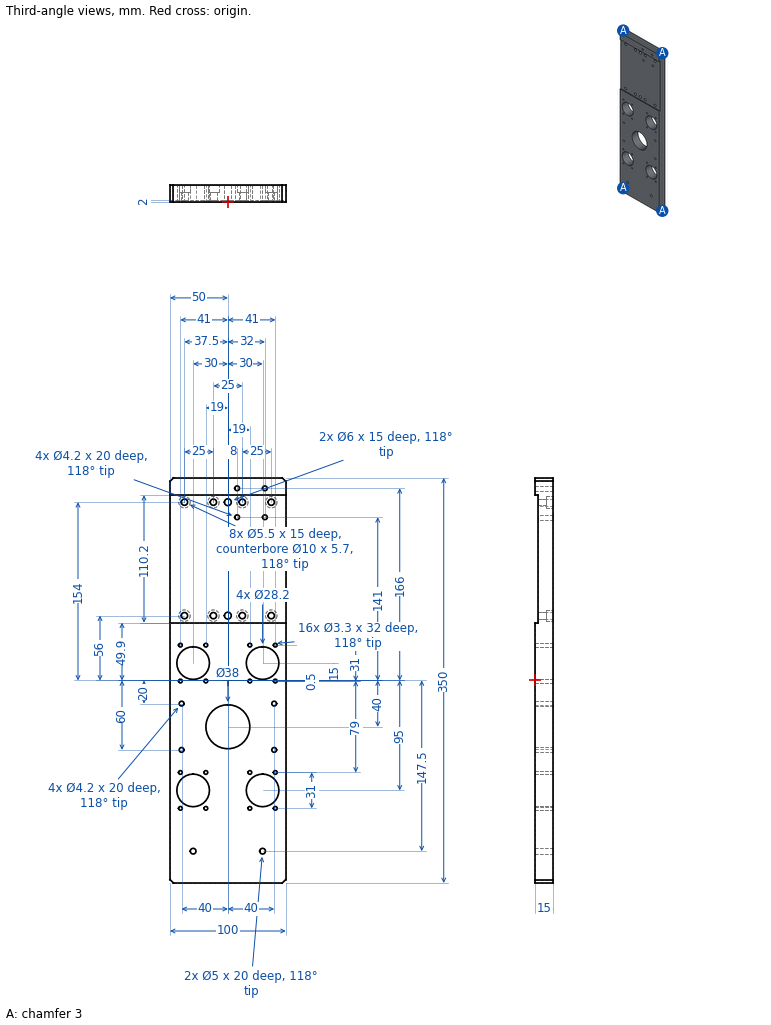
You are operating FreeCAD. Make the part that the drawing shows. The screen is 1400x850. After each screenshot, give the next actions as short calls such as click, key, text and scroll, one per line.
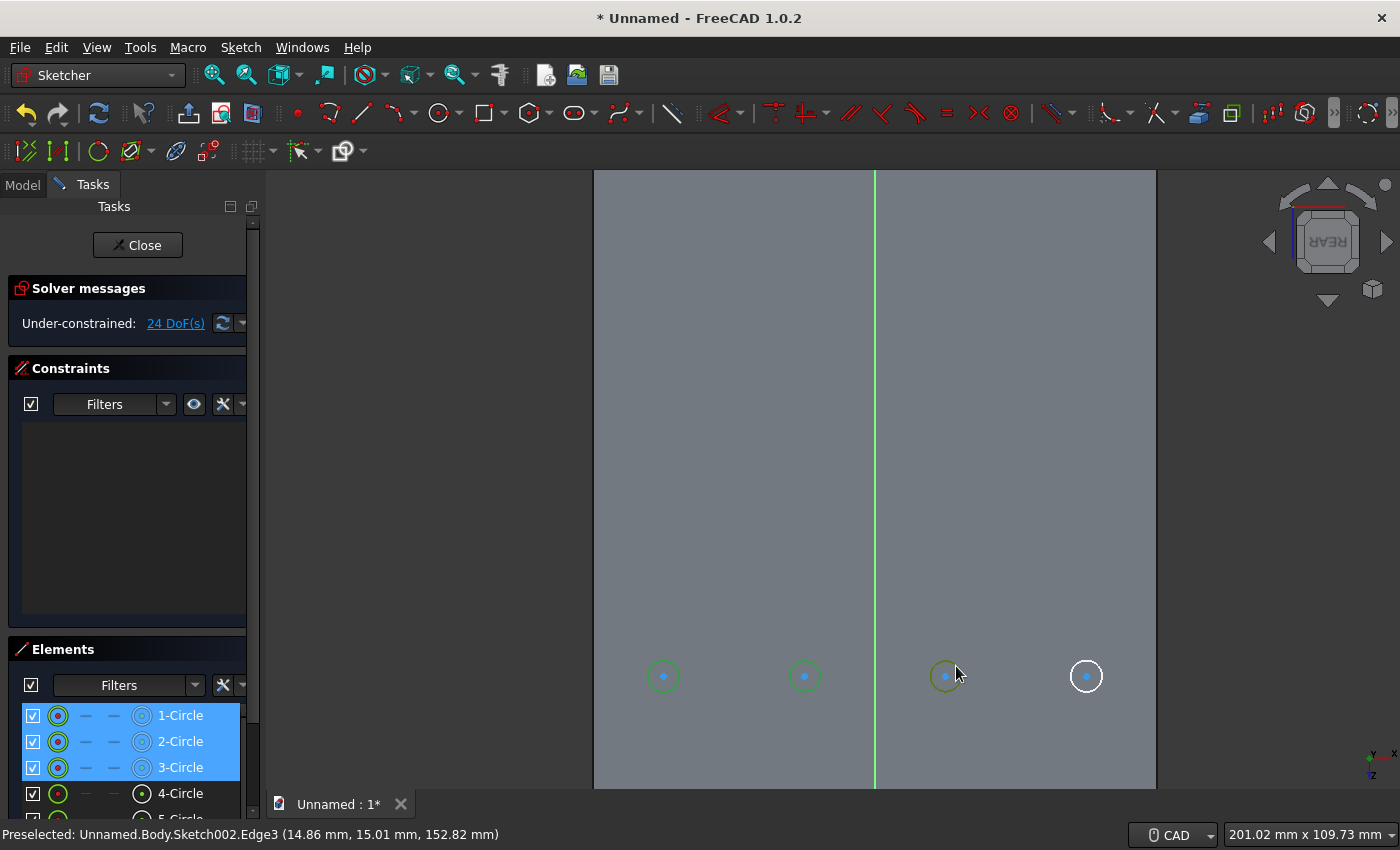
click(1097, 665)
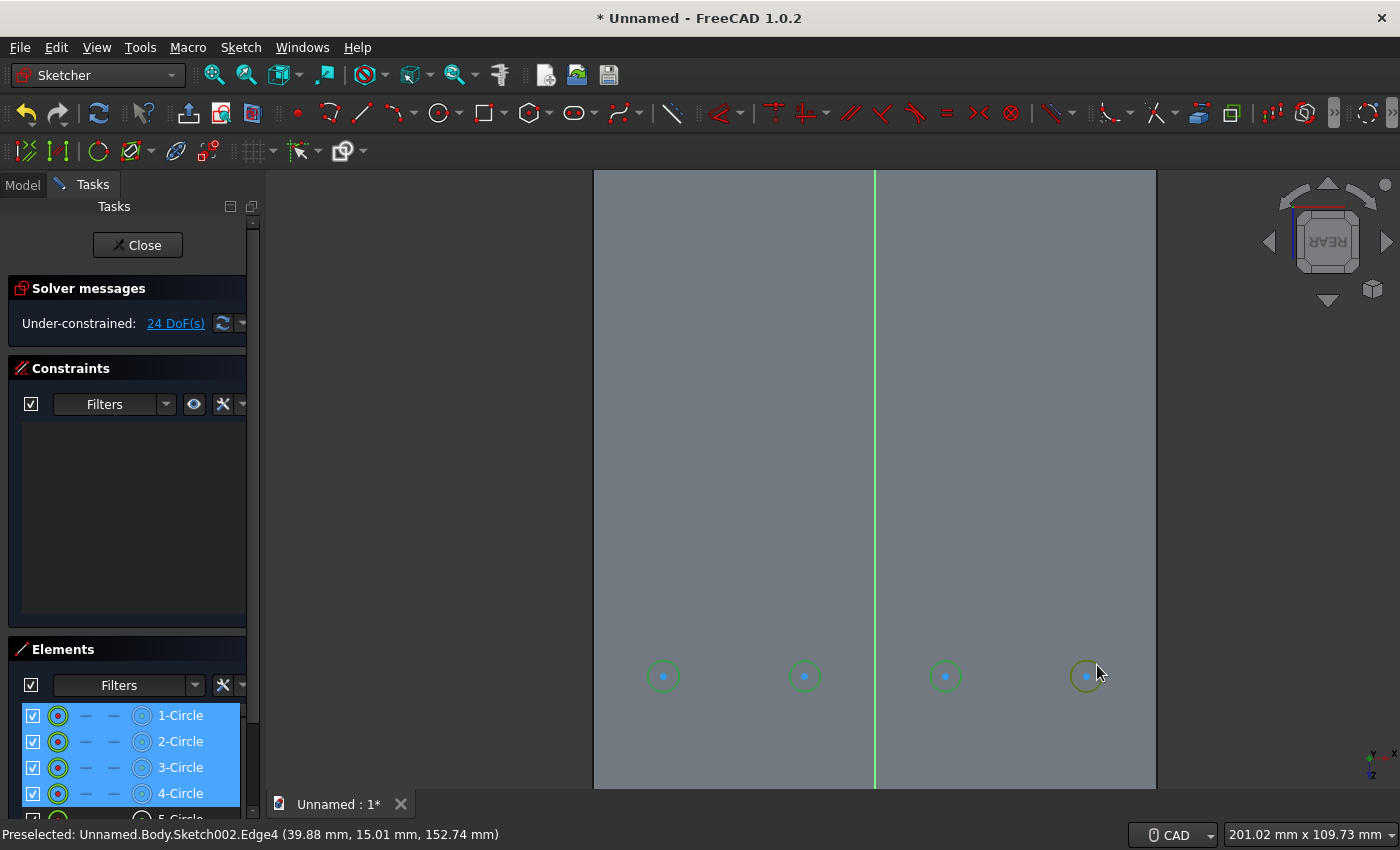
scroll(674, 667, down, 4)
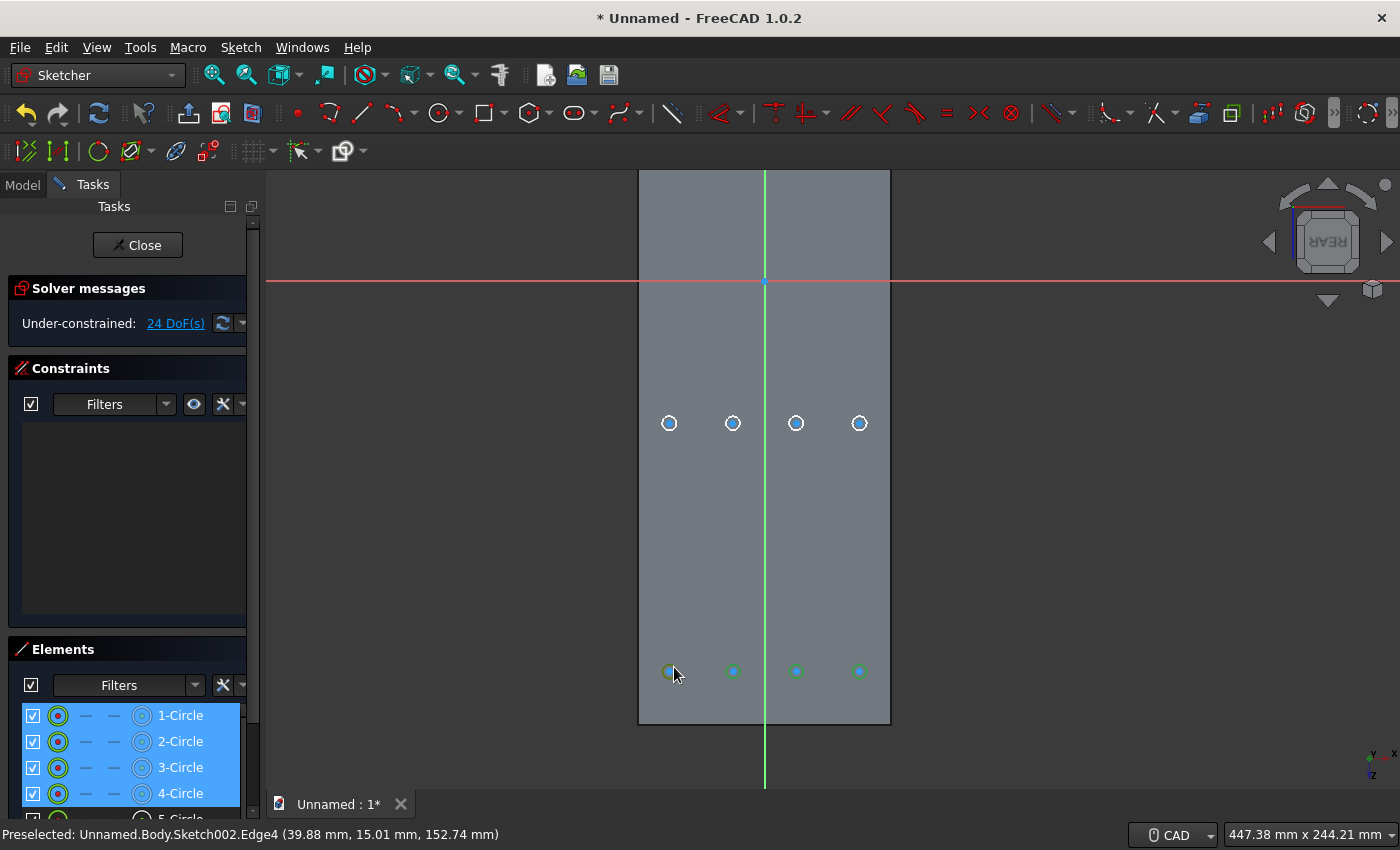
scroll(674, 418, up, 4)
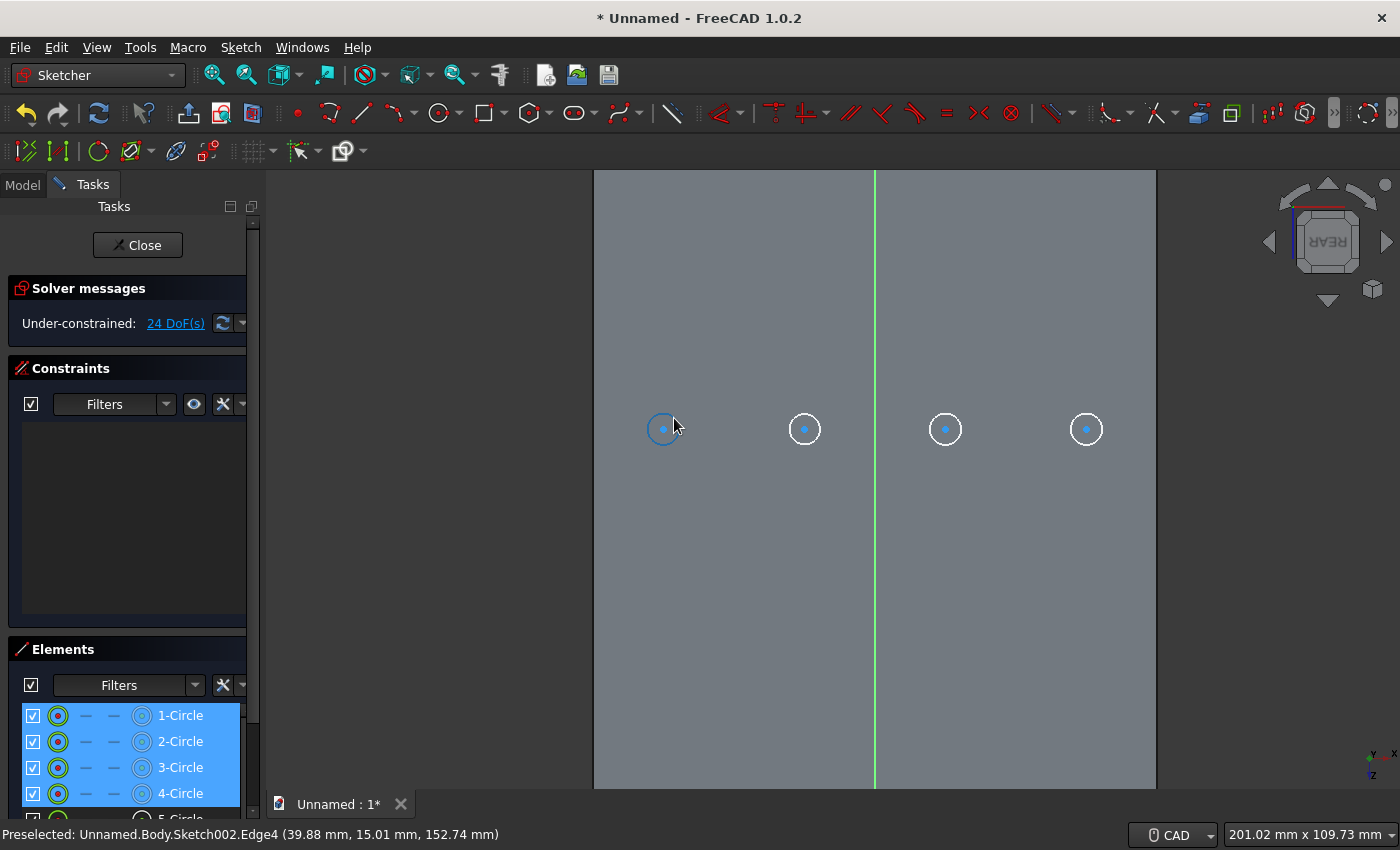
click(674, 418)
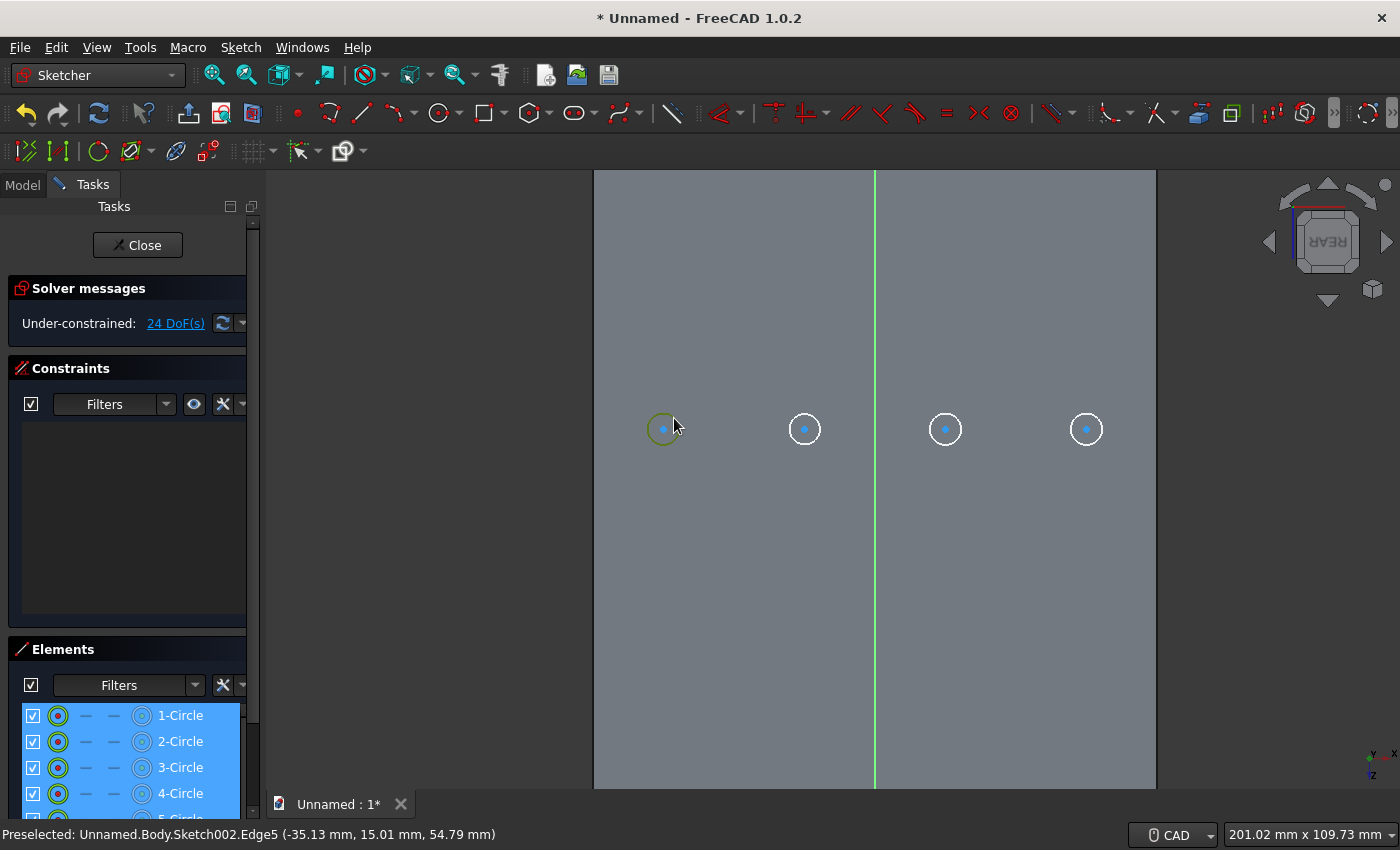
click(815, 419)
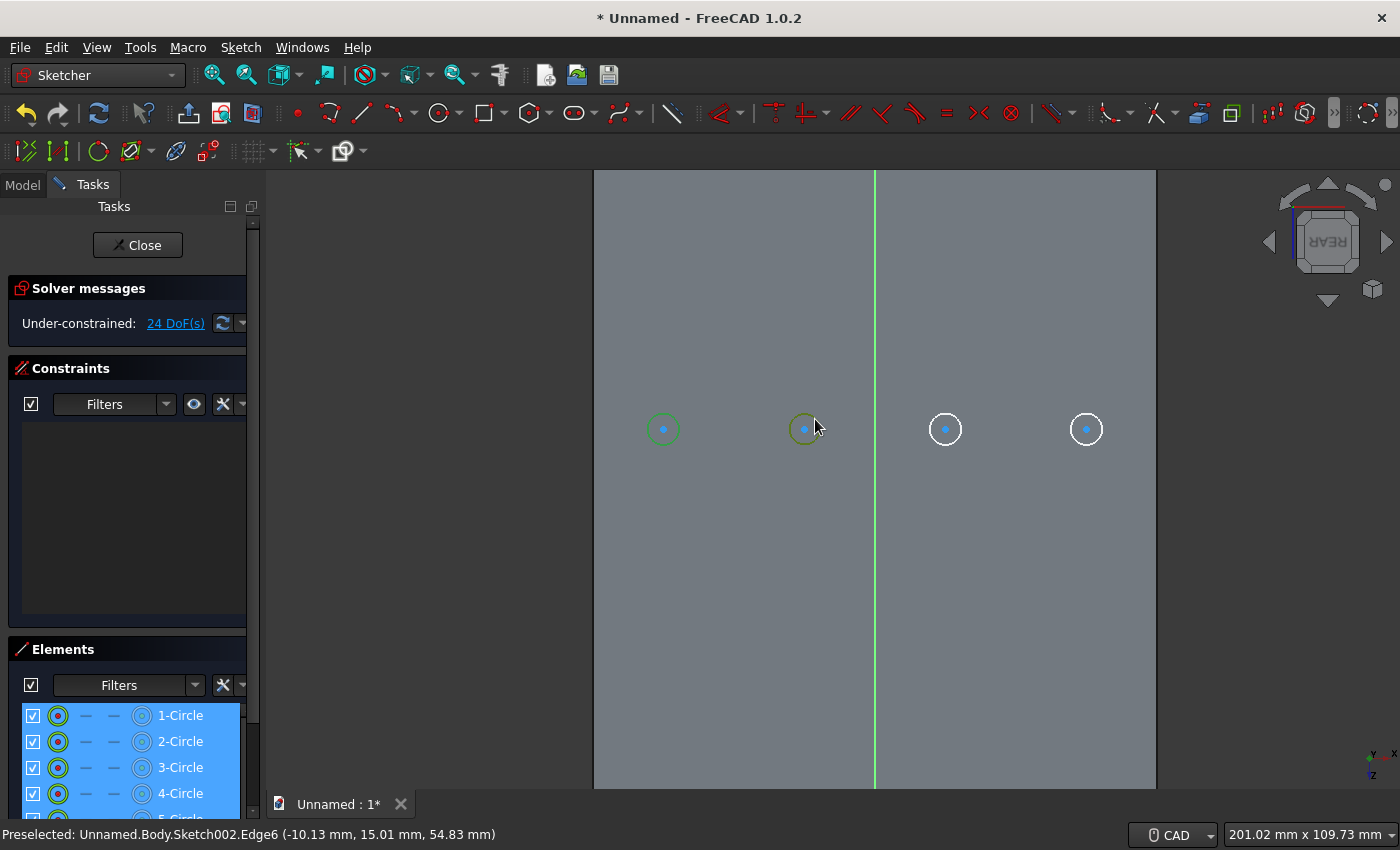
click(957, 418)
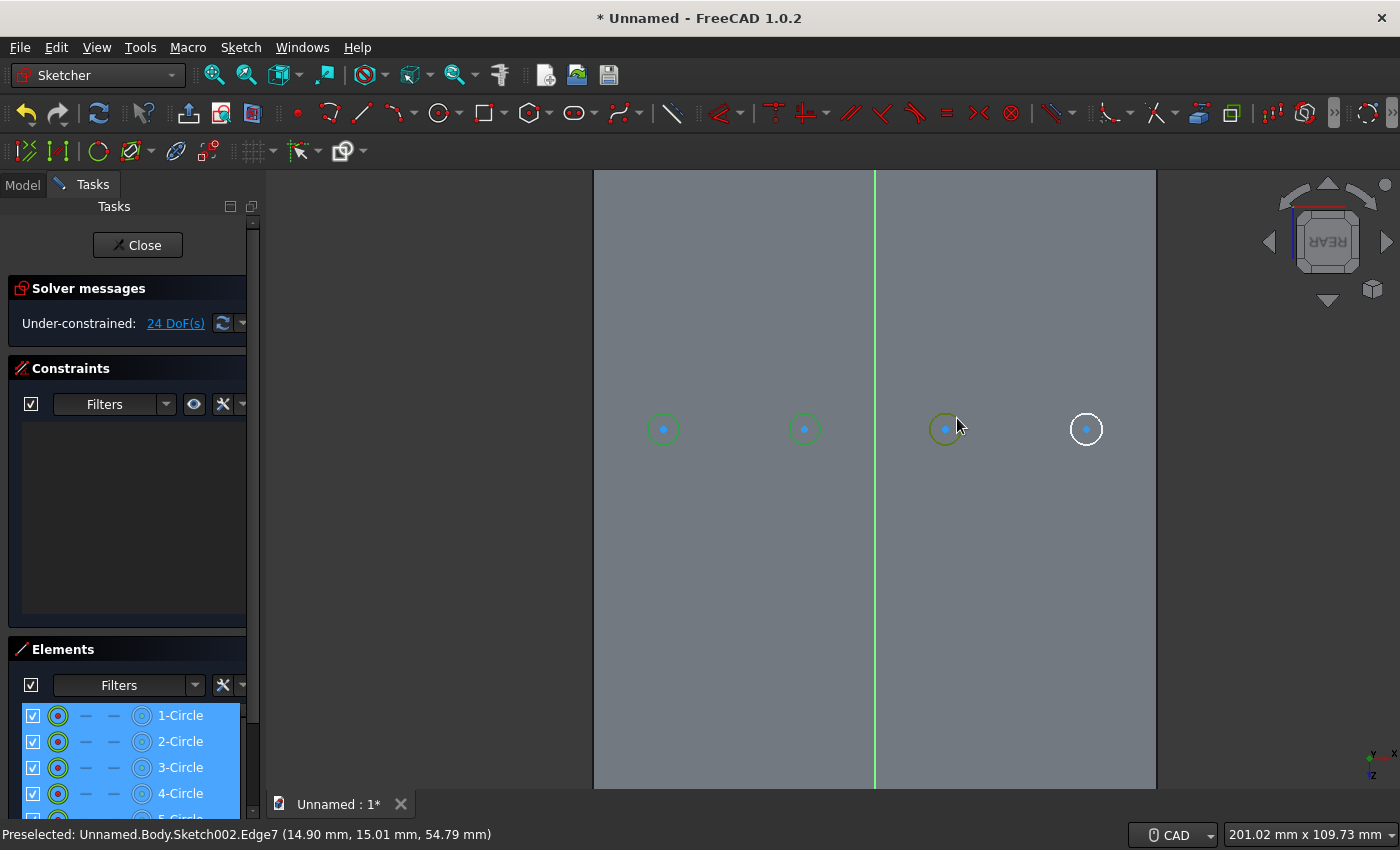
click(1097, 418)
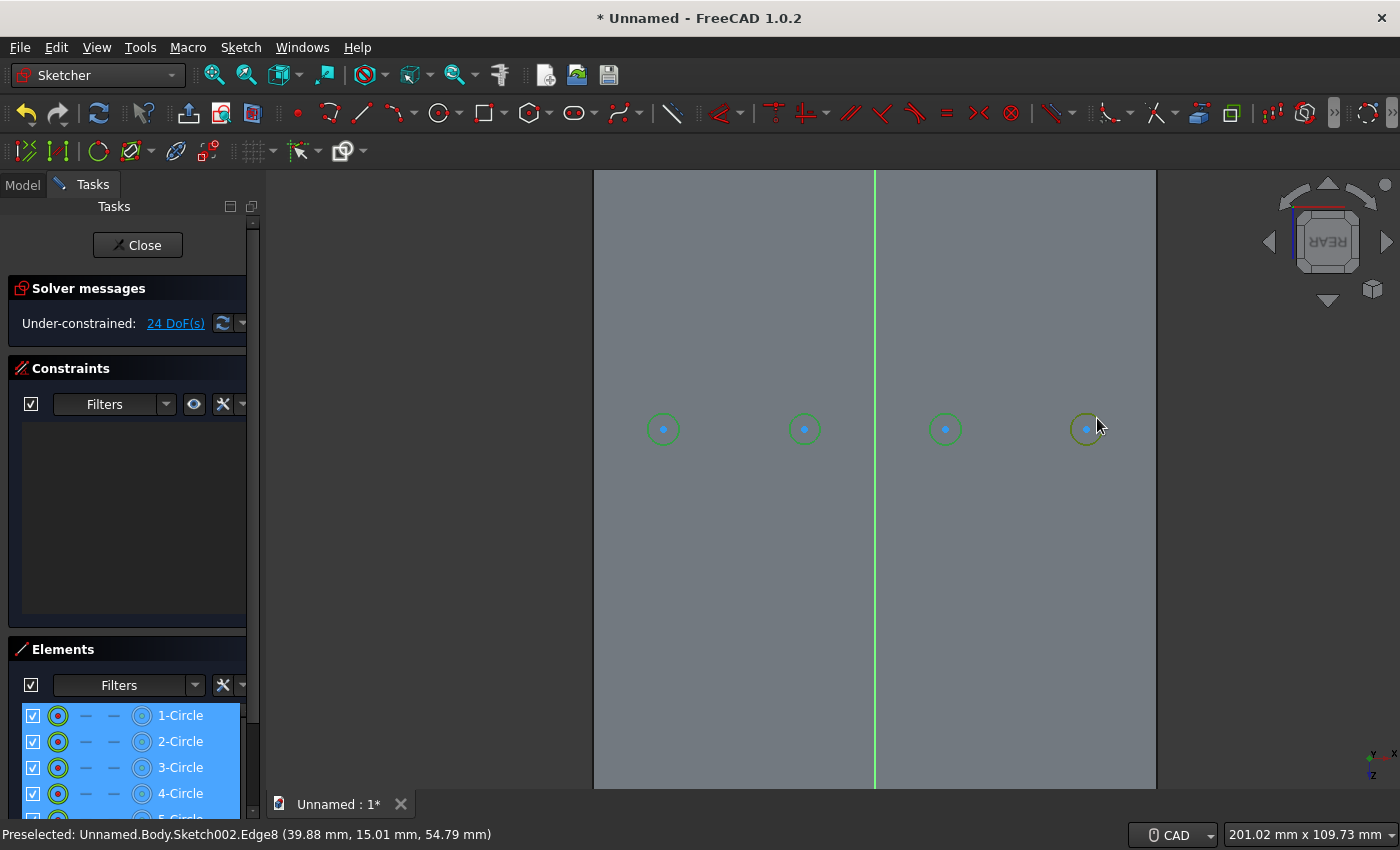
key(e)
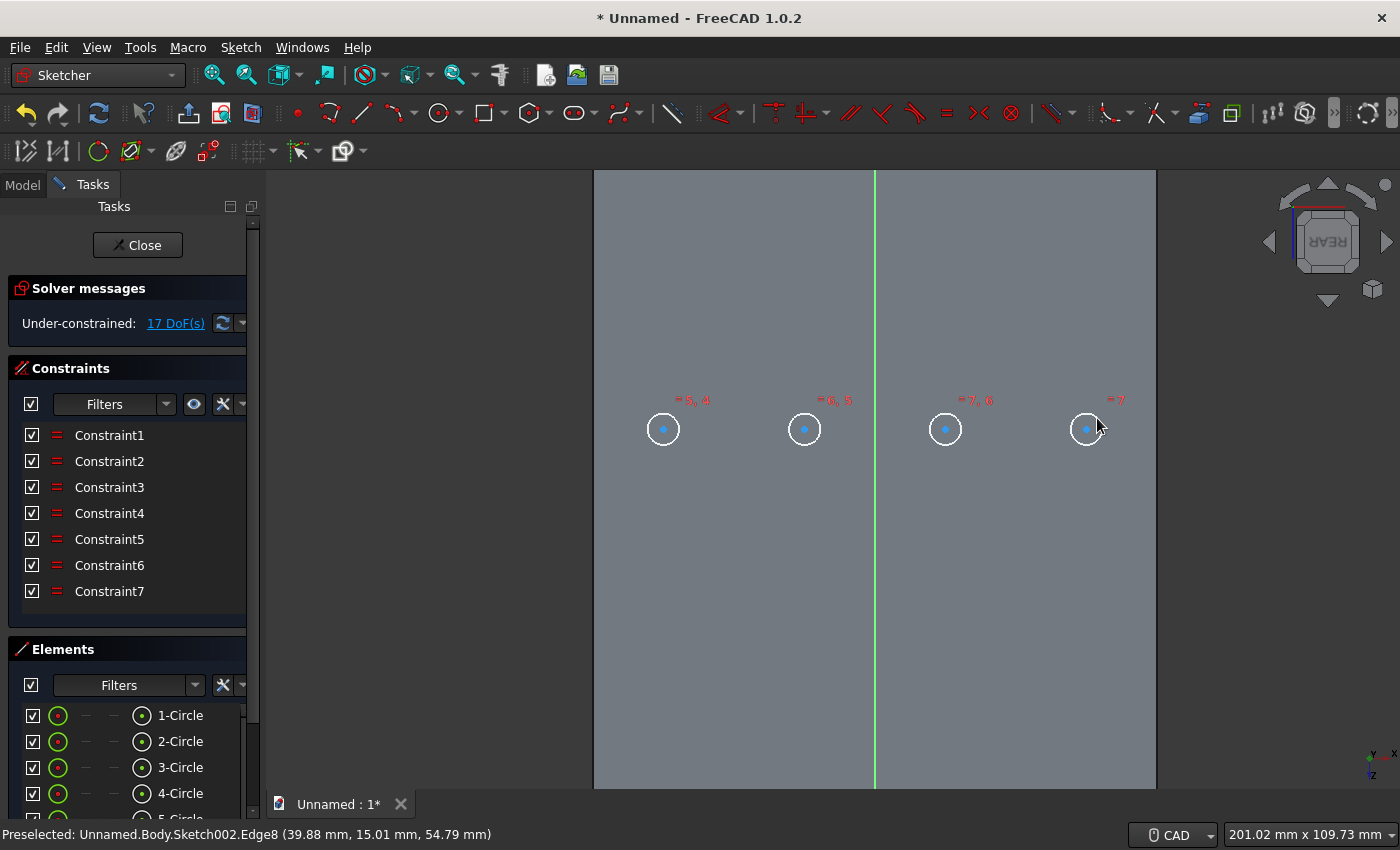
scroll(674, 418, down, 4)